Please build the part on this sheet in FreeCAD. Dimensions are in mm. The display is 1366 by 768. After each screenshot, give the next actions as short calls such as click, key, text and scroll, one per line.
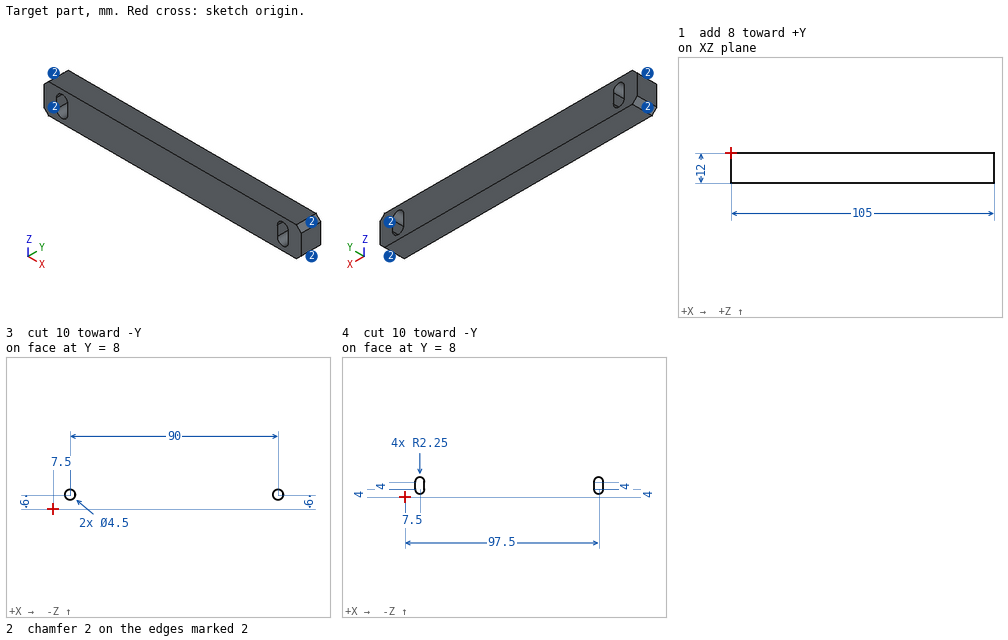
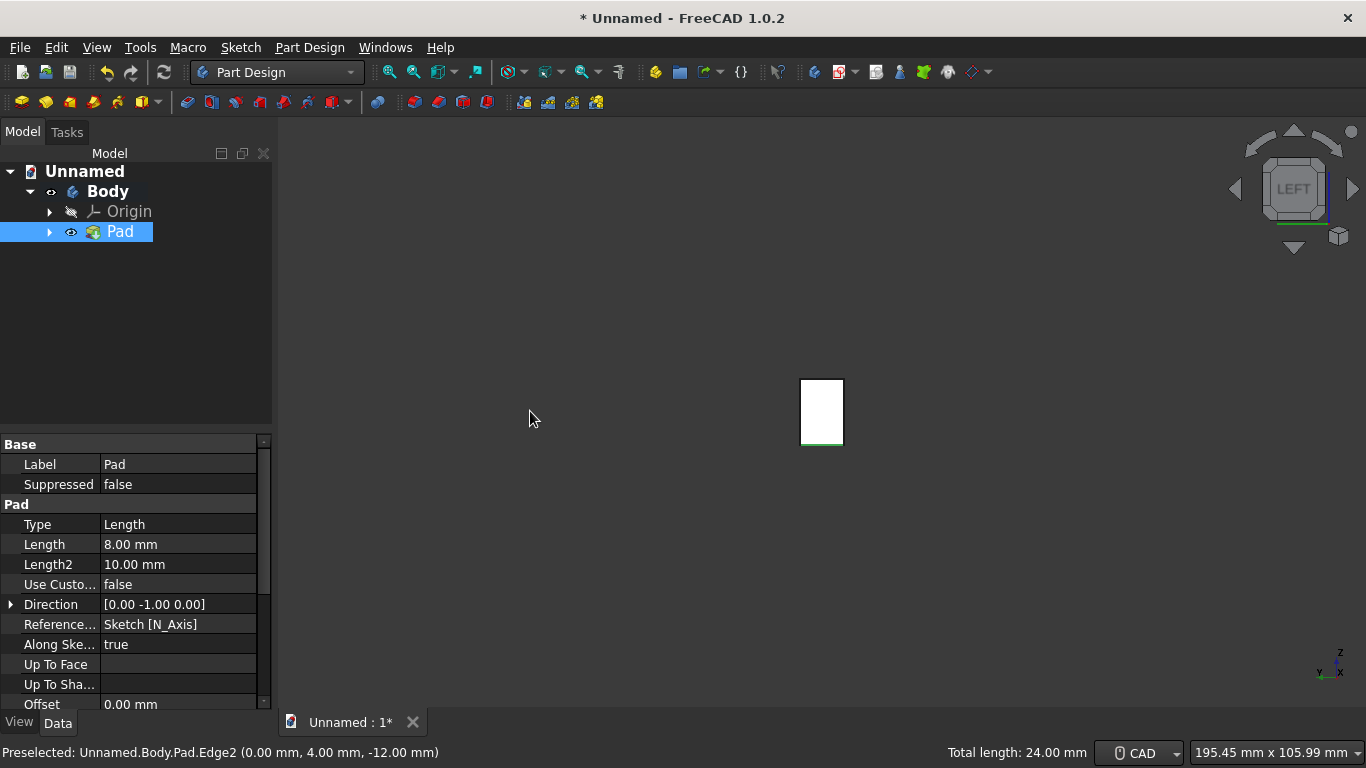
click(390, 72)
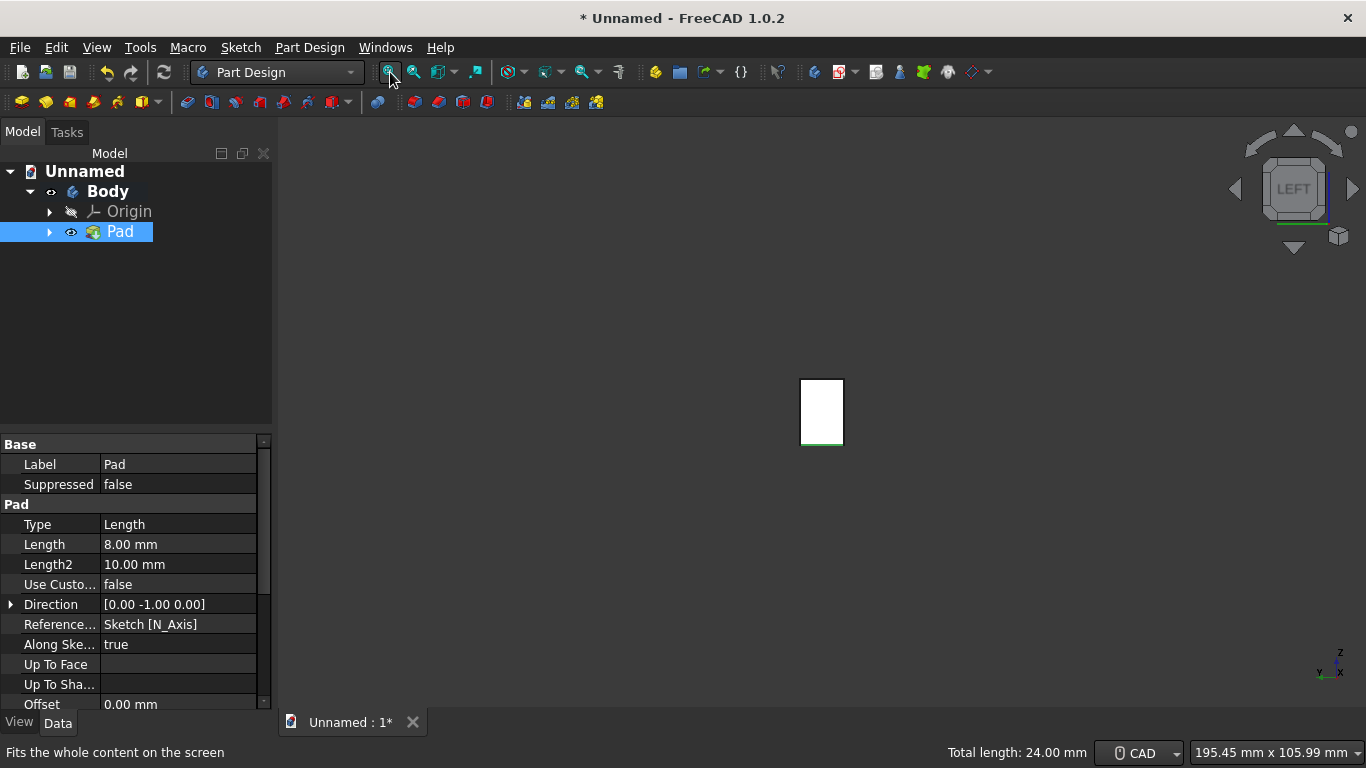
click(822, 378, ctrl)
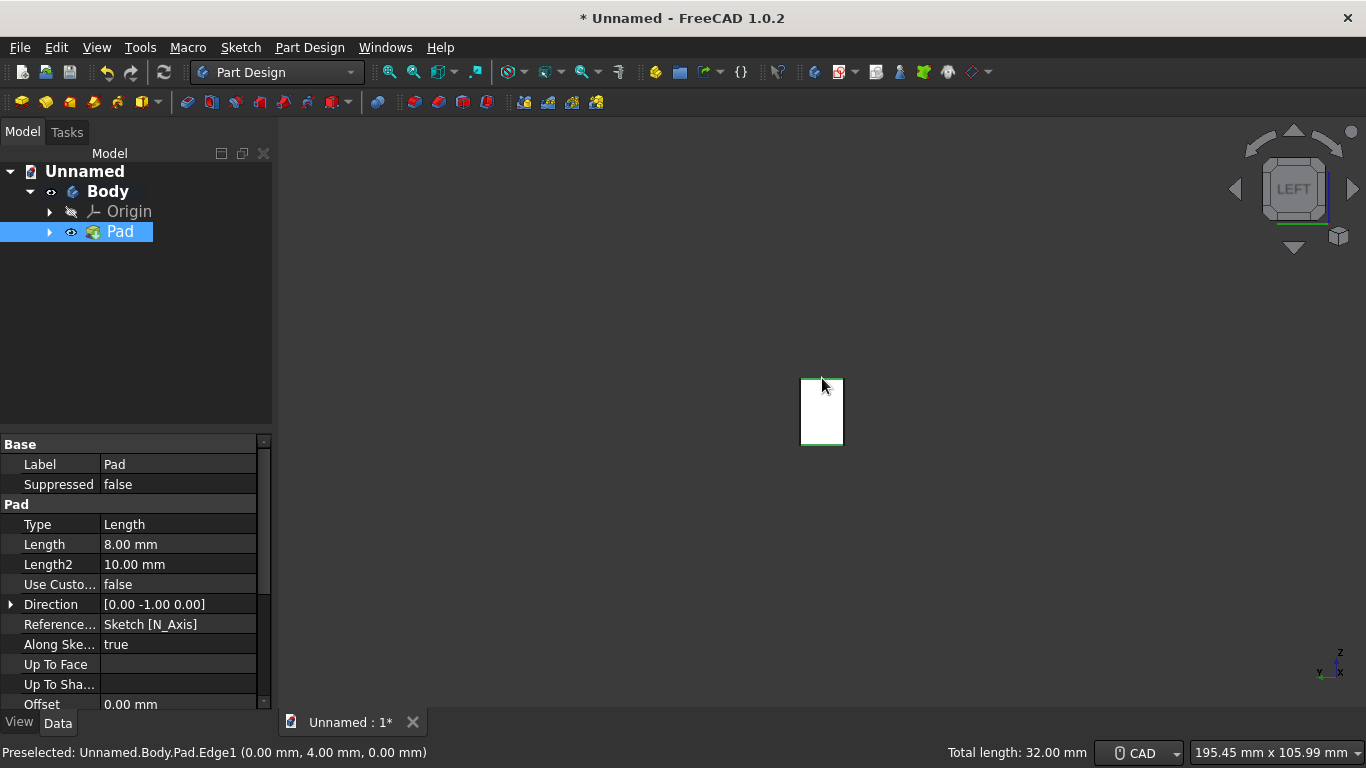
click(440, 102)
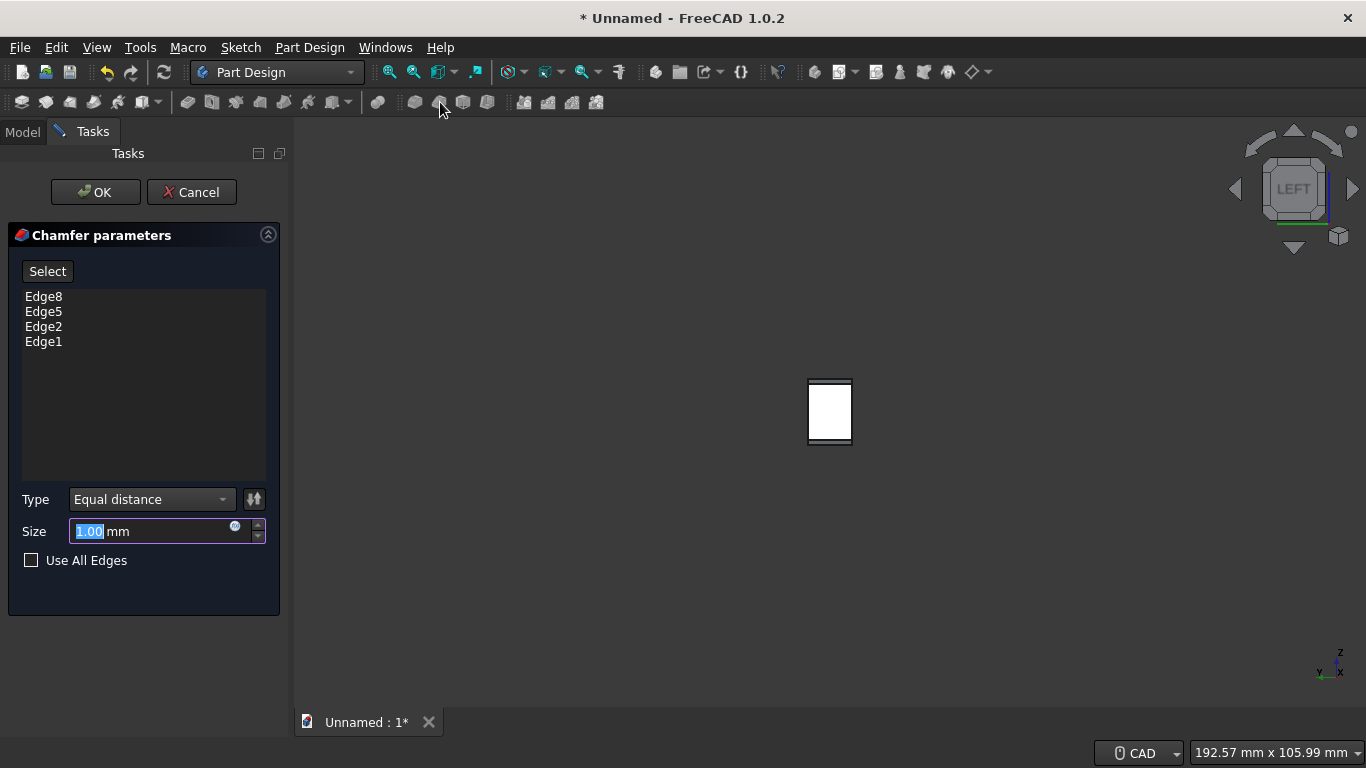
text(2)
key(Tab)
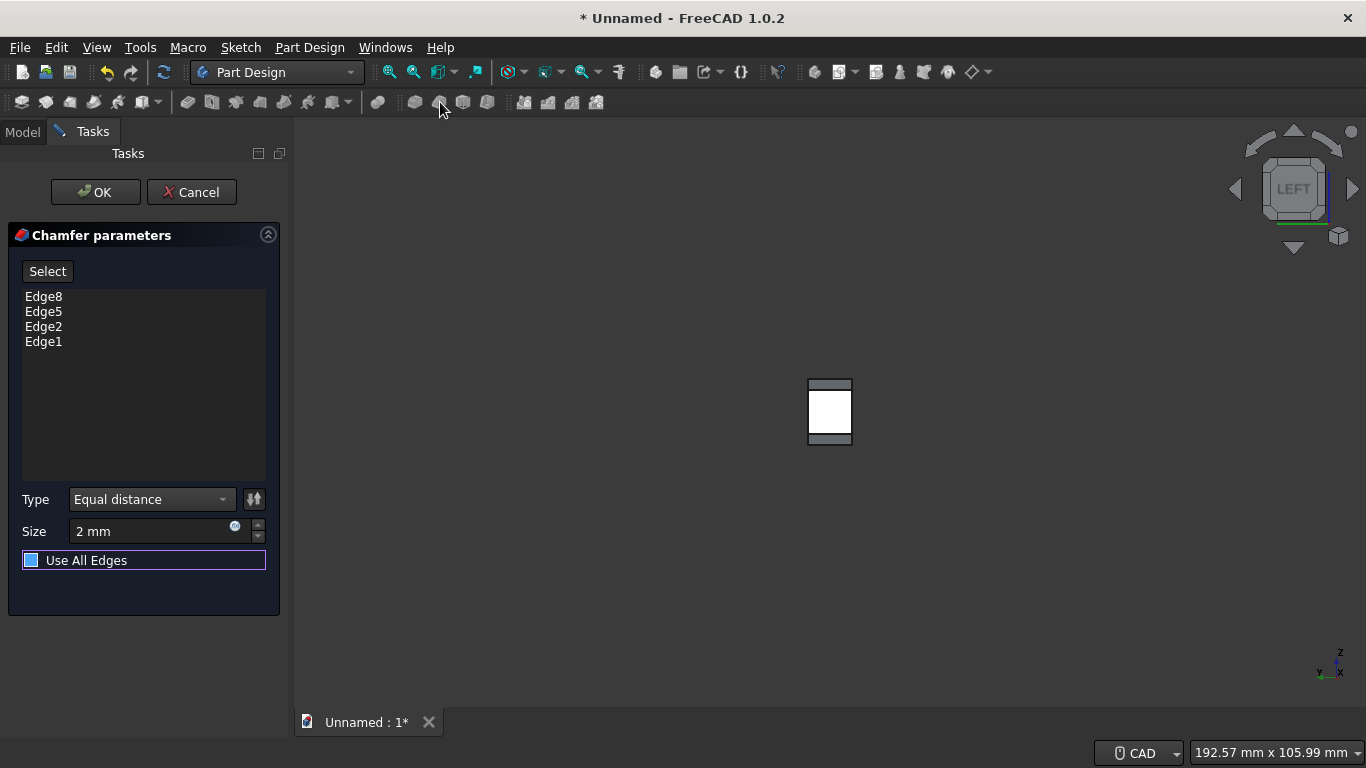
click(96, 192)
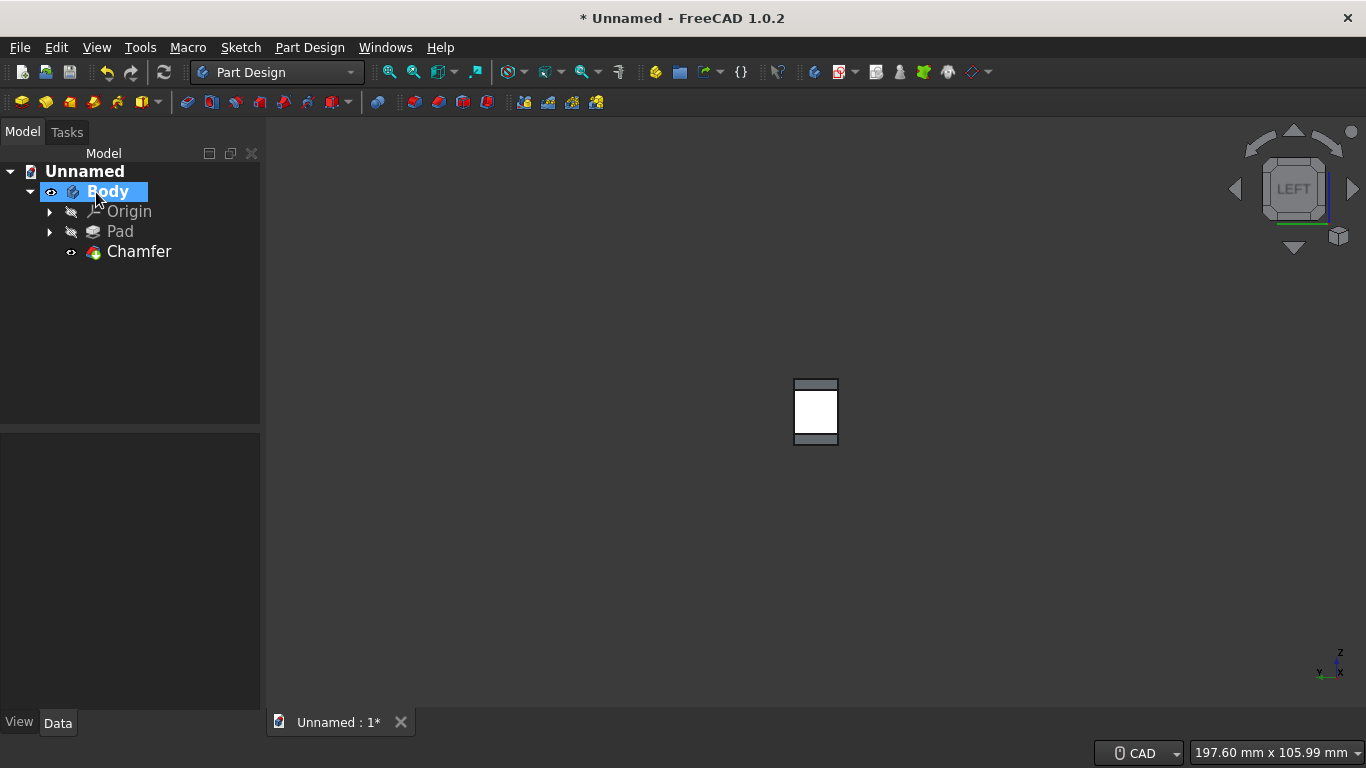
click(390, 72)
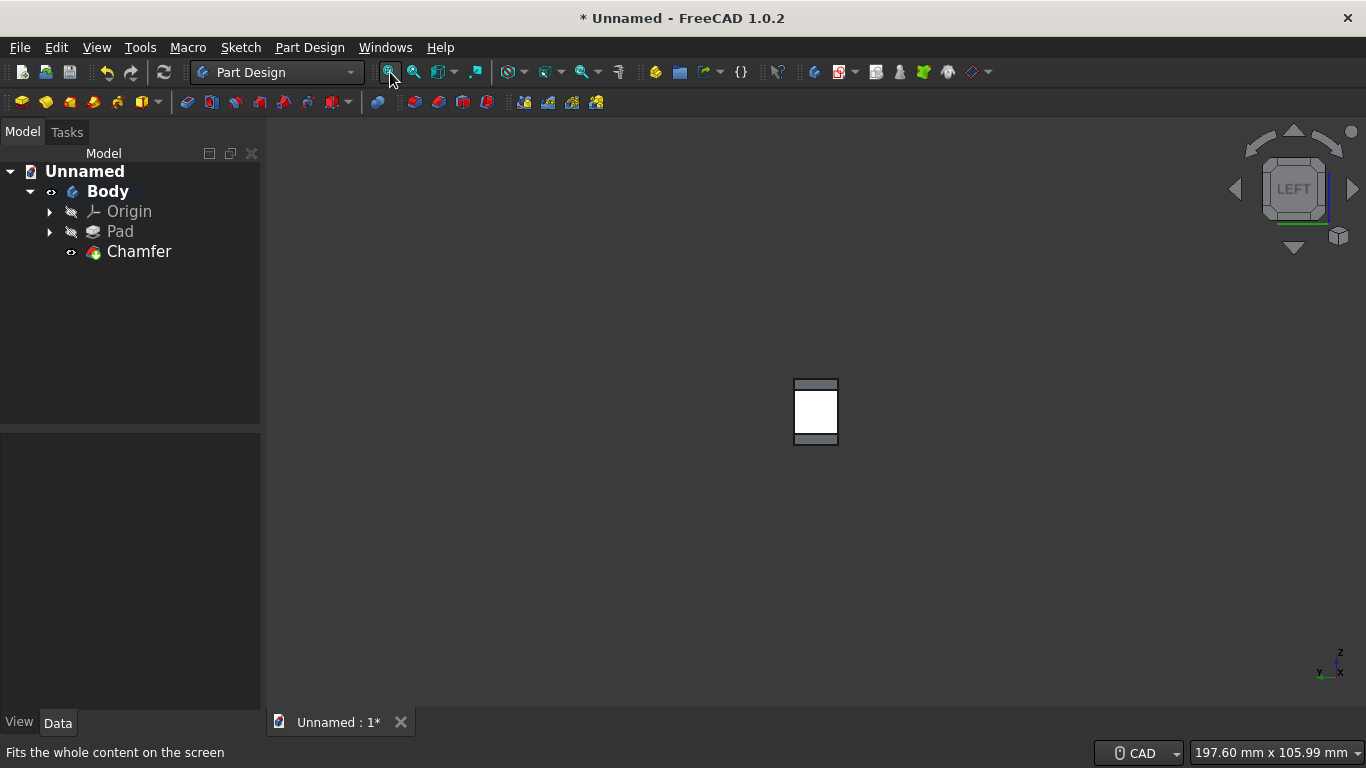
key(4)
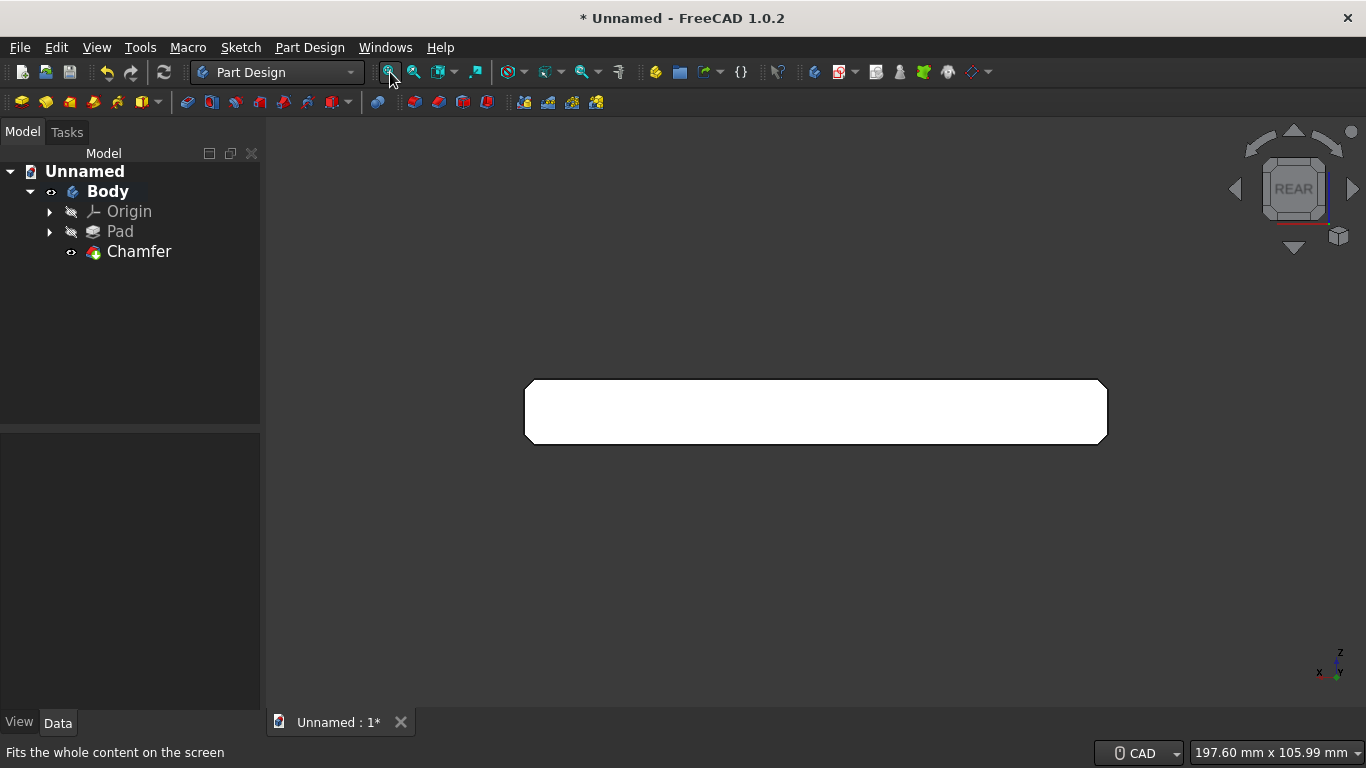
click(565, 411)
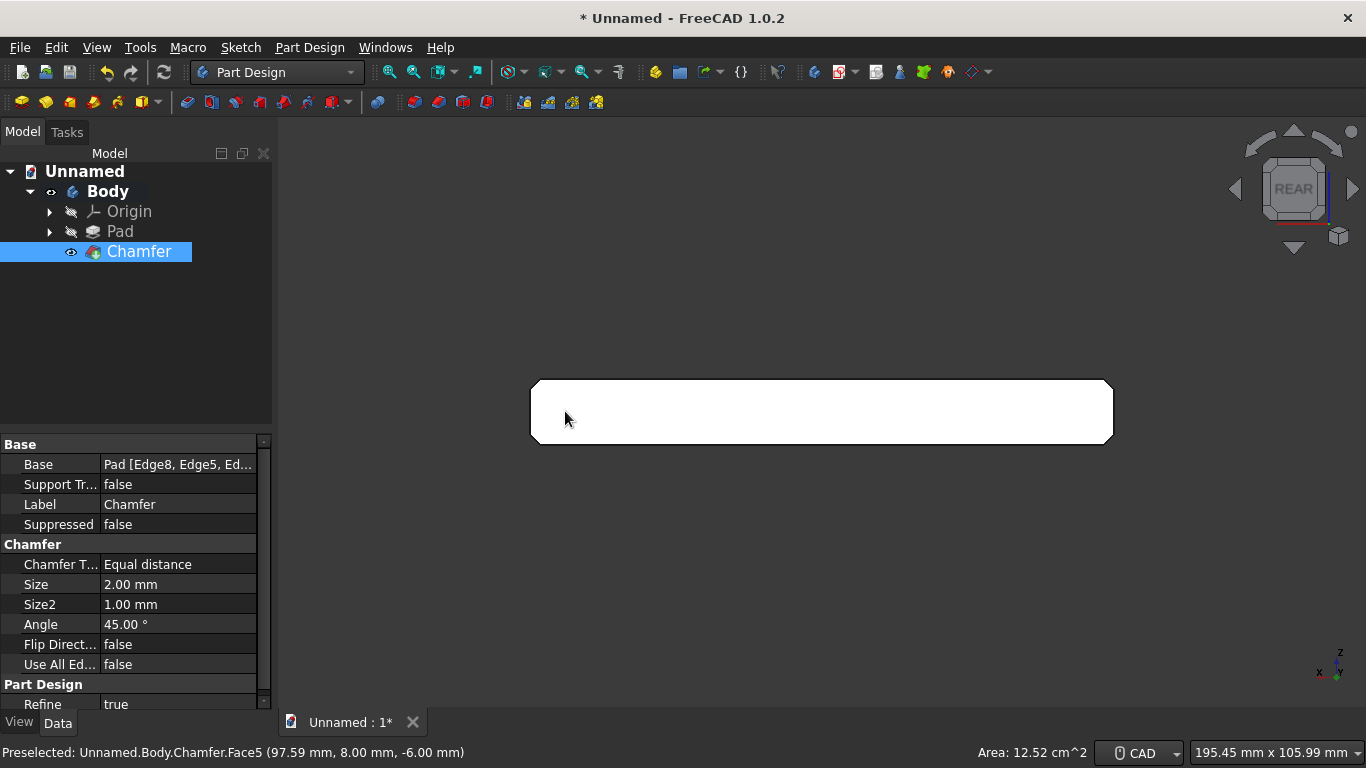
click(840, 72)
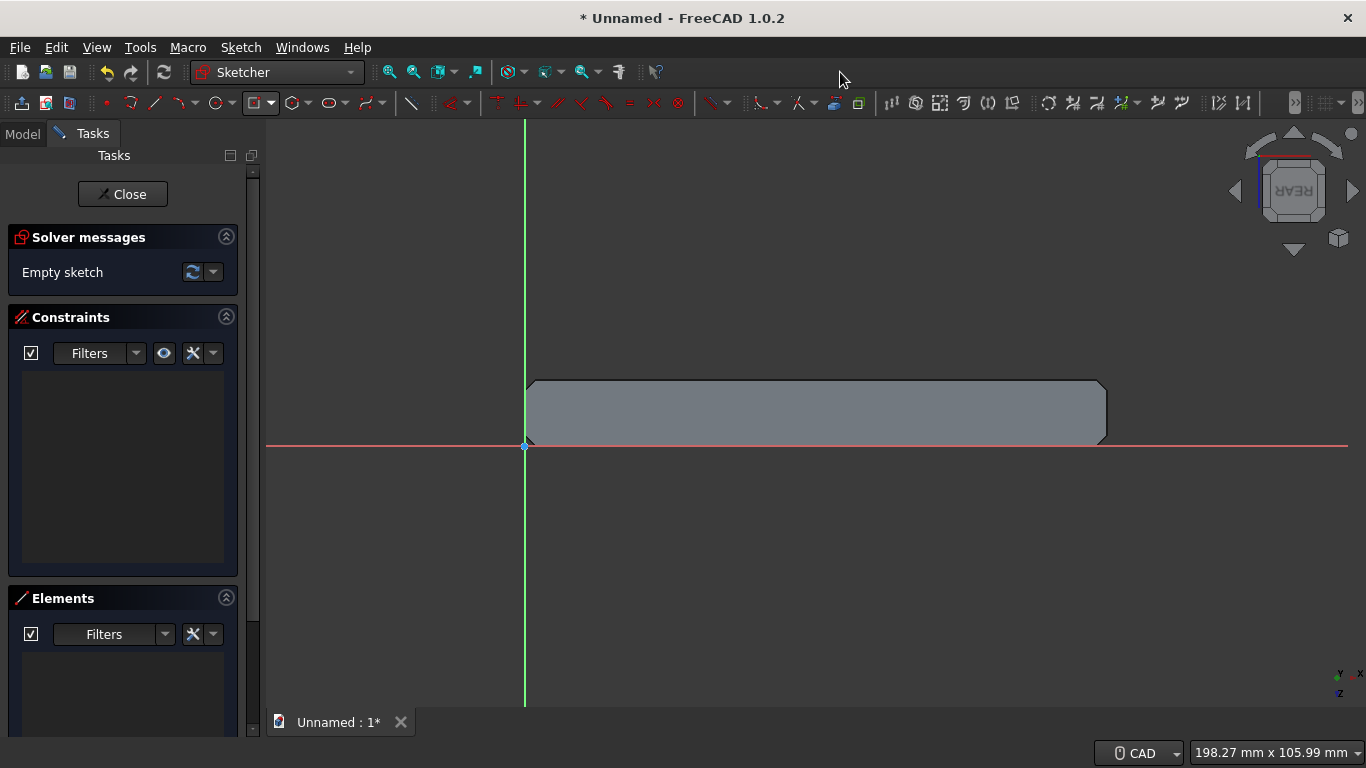
click(216, 104)